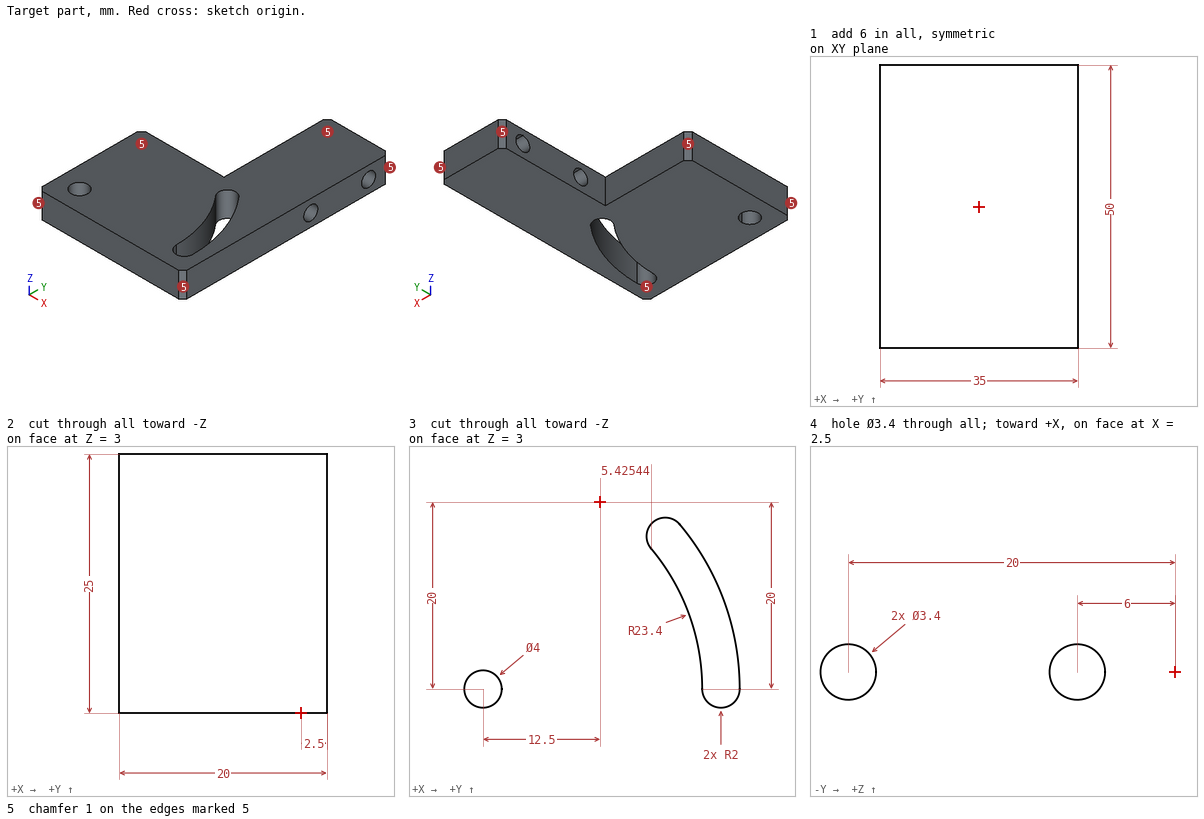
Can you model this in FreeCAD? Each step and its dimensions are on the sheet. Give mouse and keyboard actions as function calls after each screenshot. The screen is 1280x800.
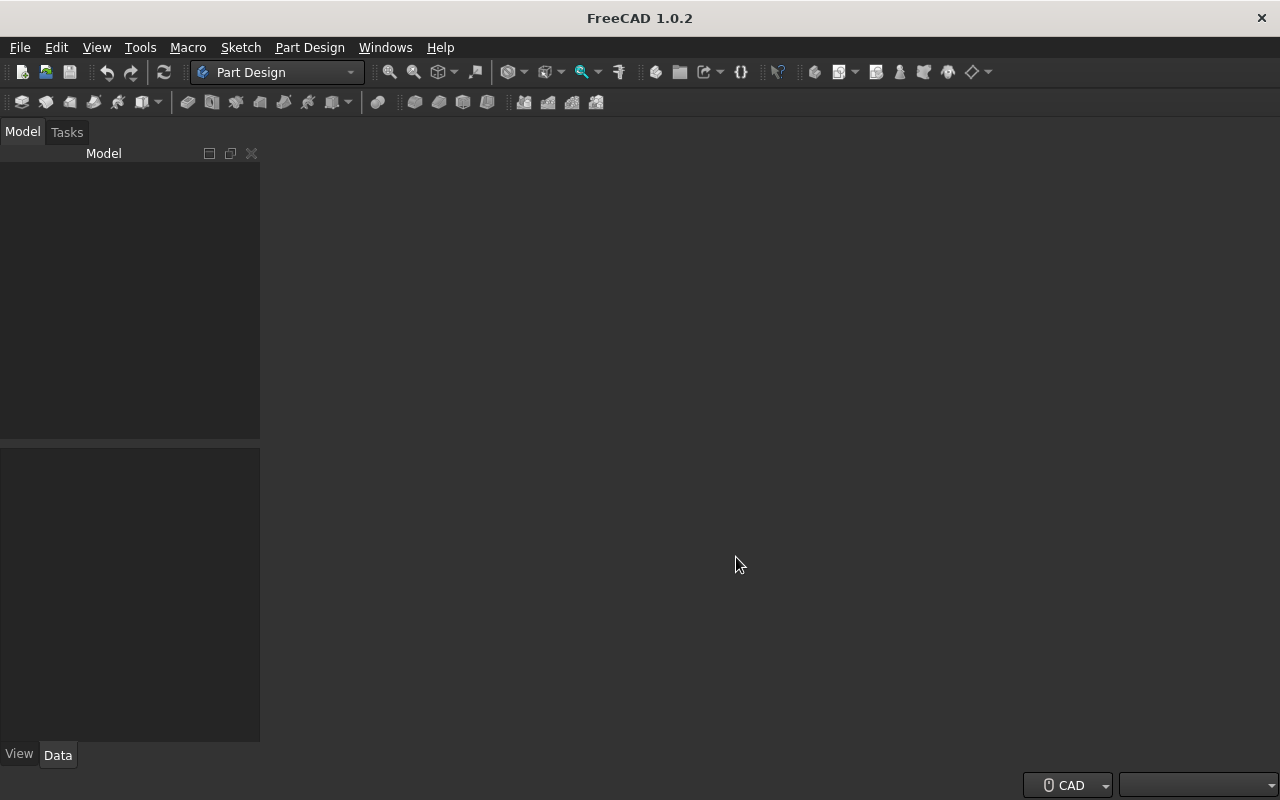
click(22, 72)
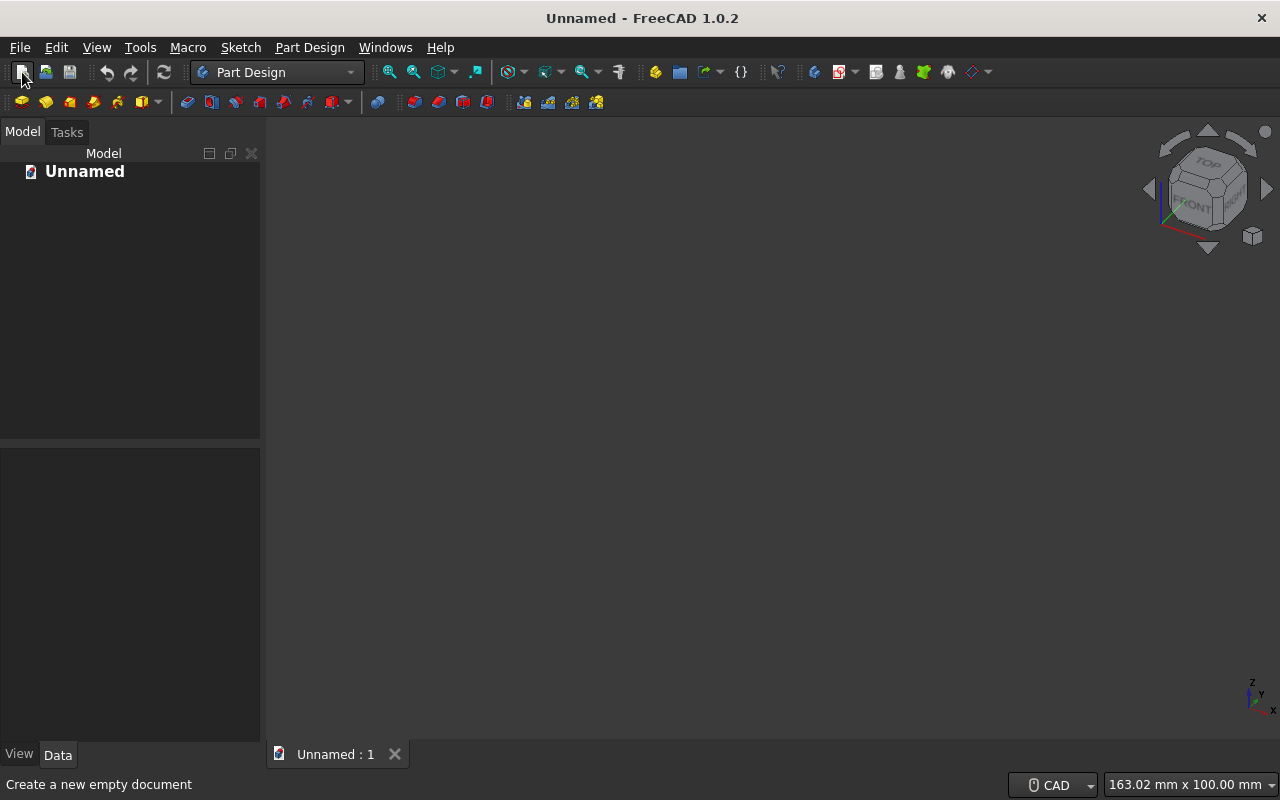
click(840, 72)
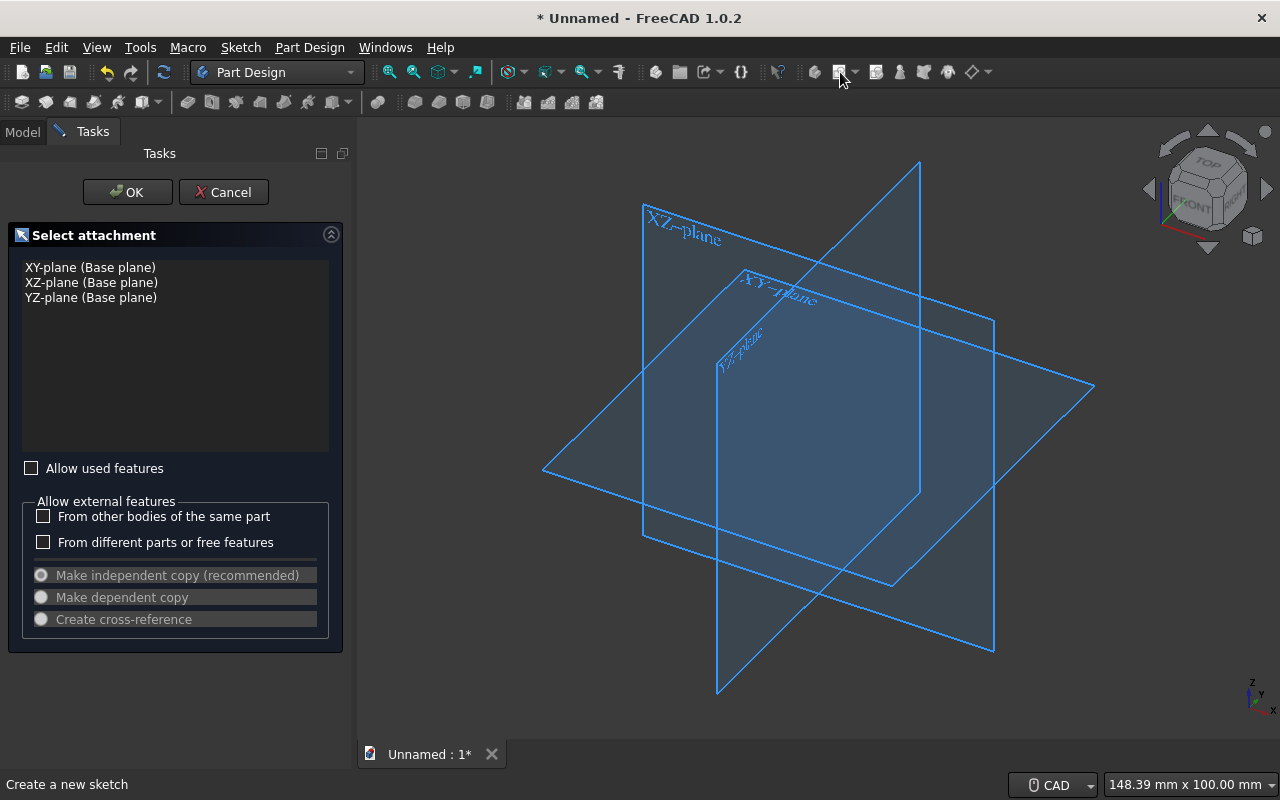
click(82, 268)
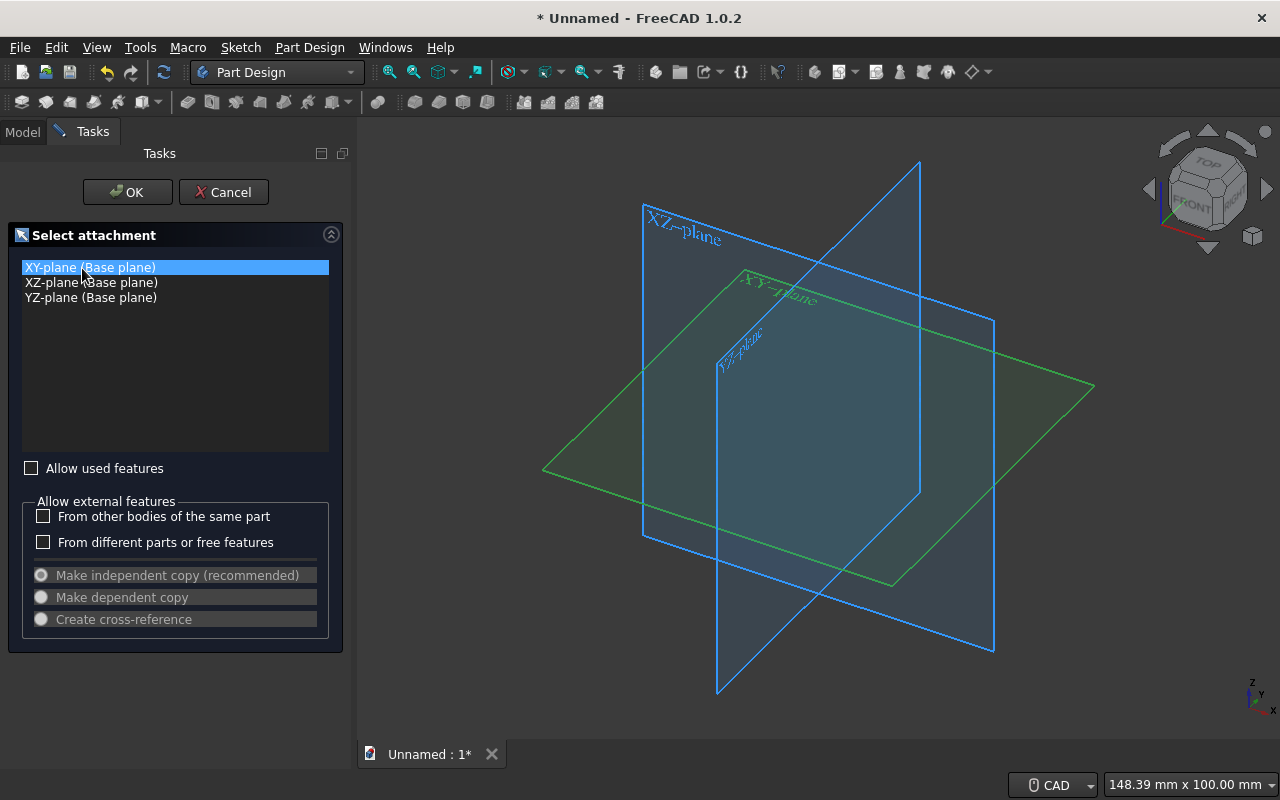
click(128, 192)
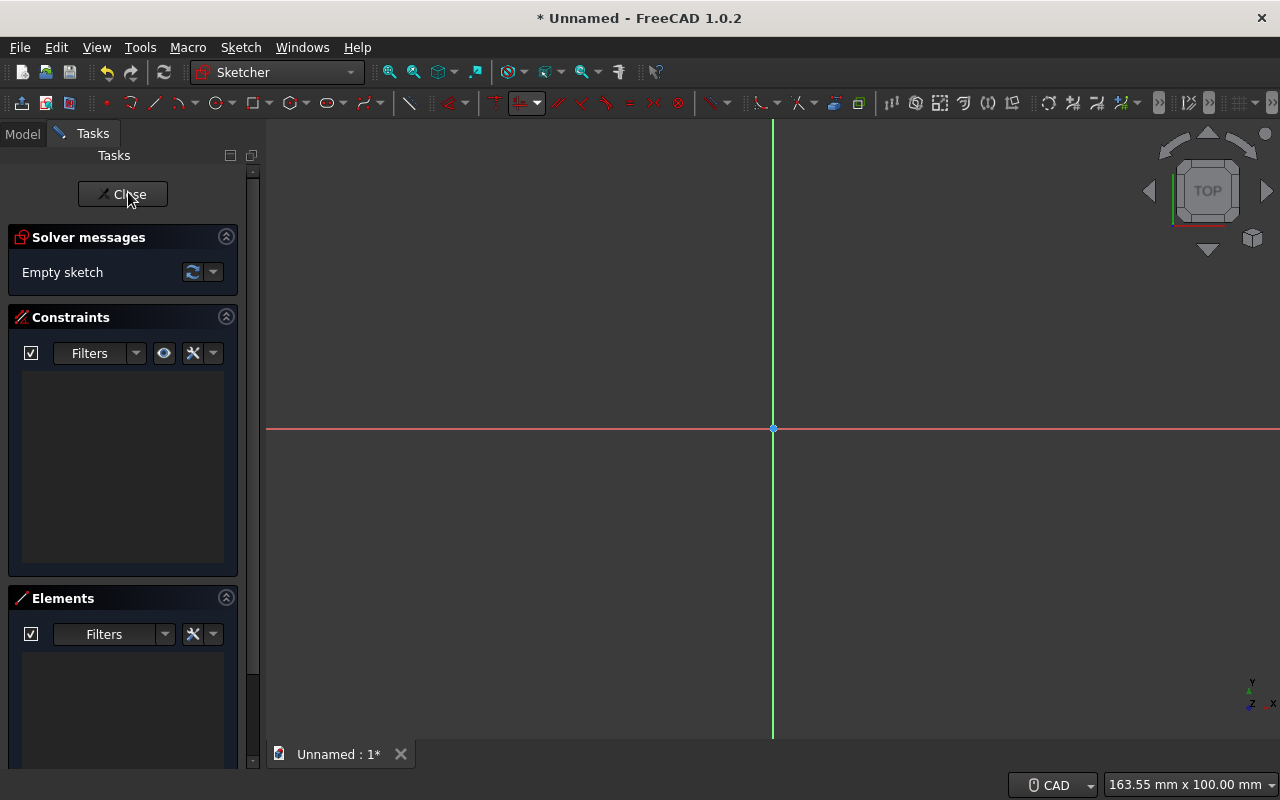
click(272, 104)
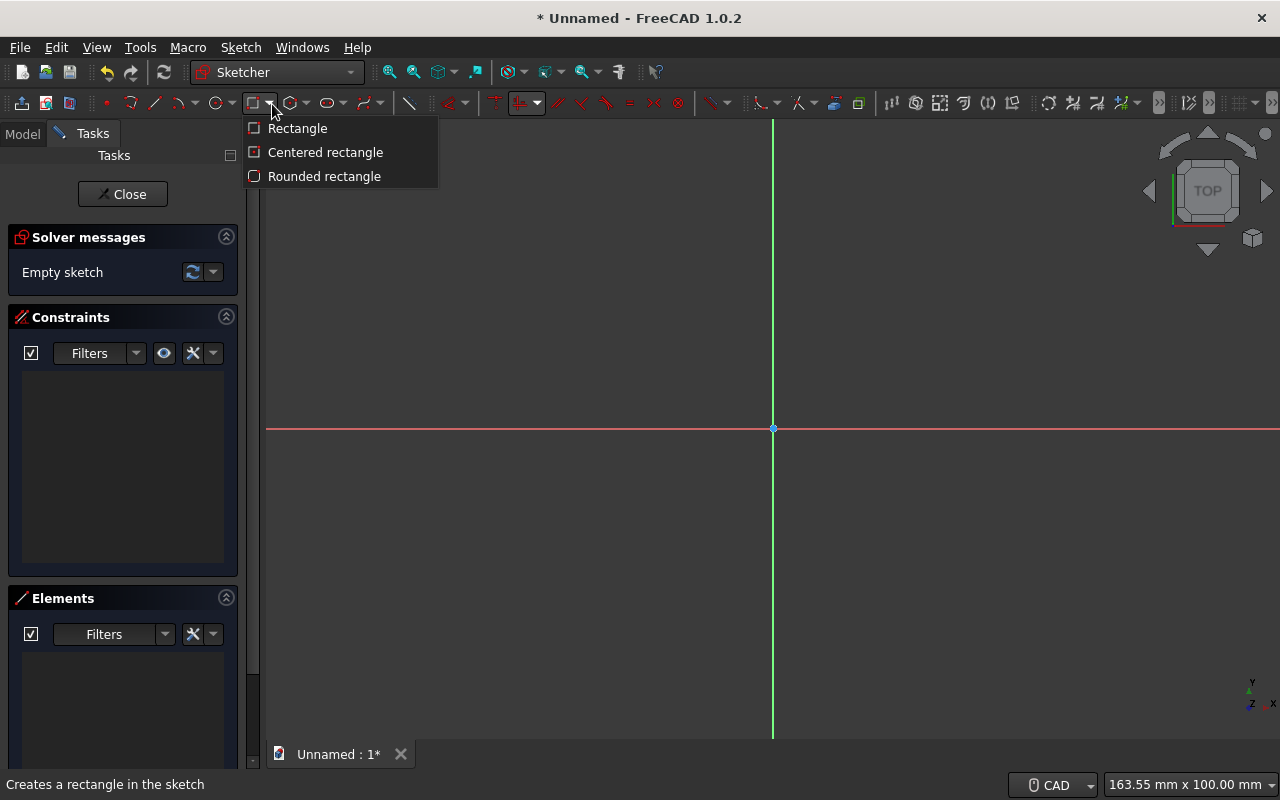
click(340, 152)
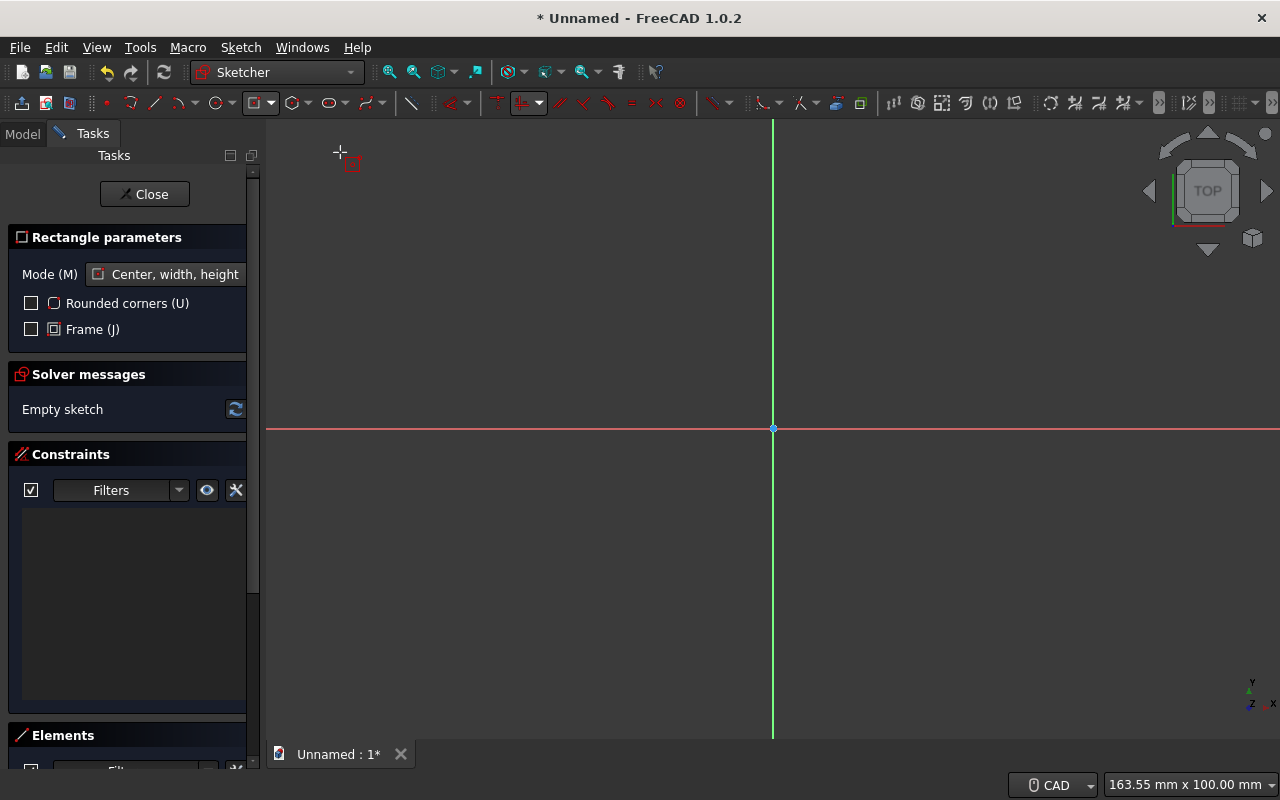
click(773, 429)
click(882, 274)
key(Escape)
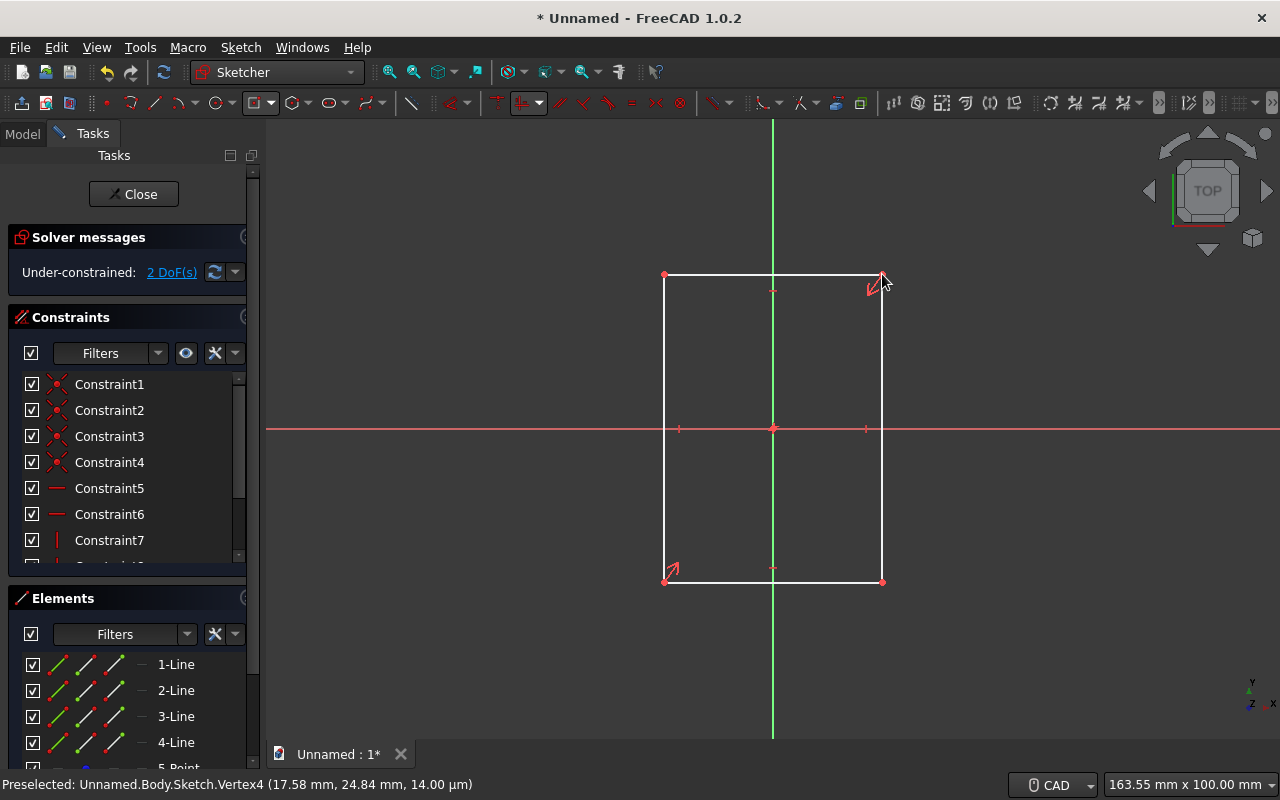
click(450, 104)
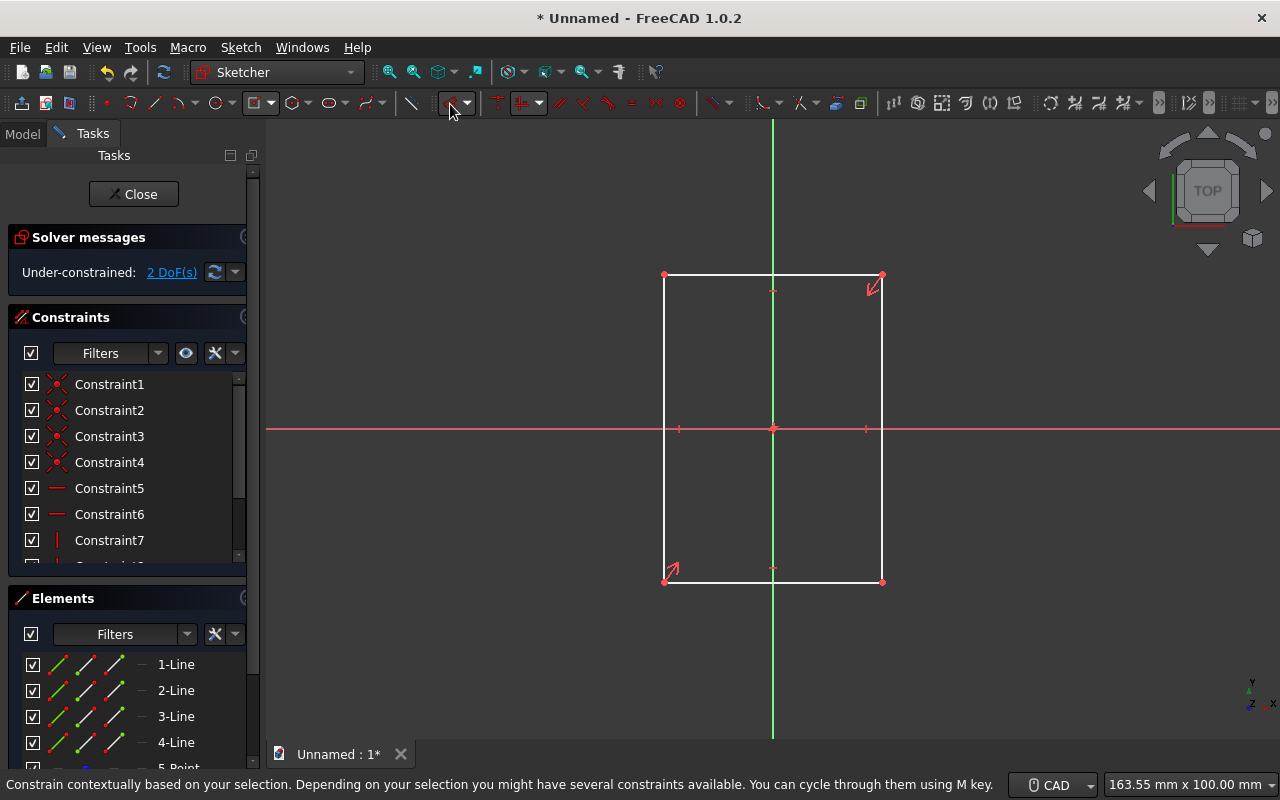
click(729, 583)
click(723, 617)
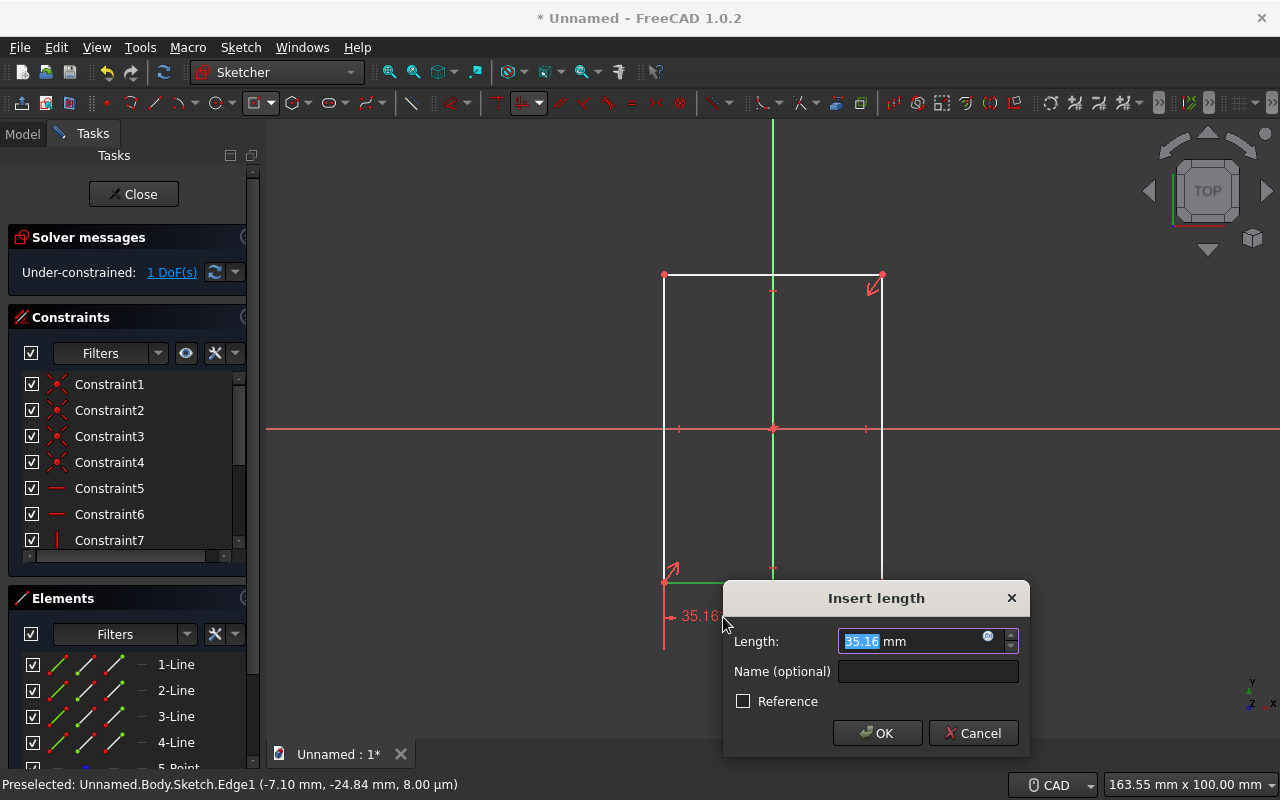
text(35)
key(Return)